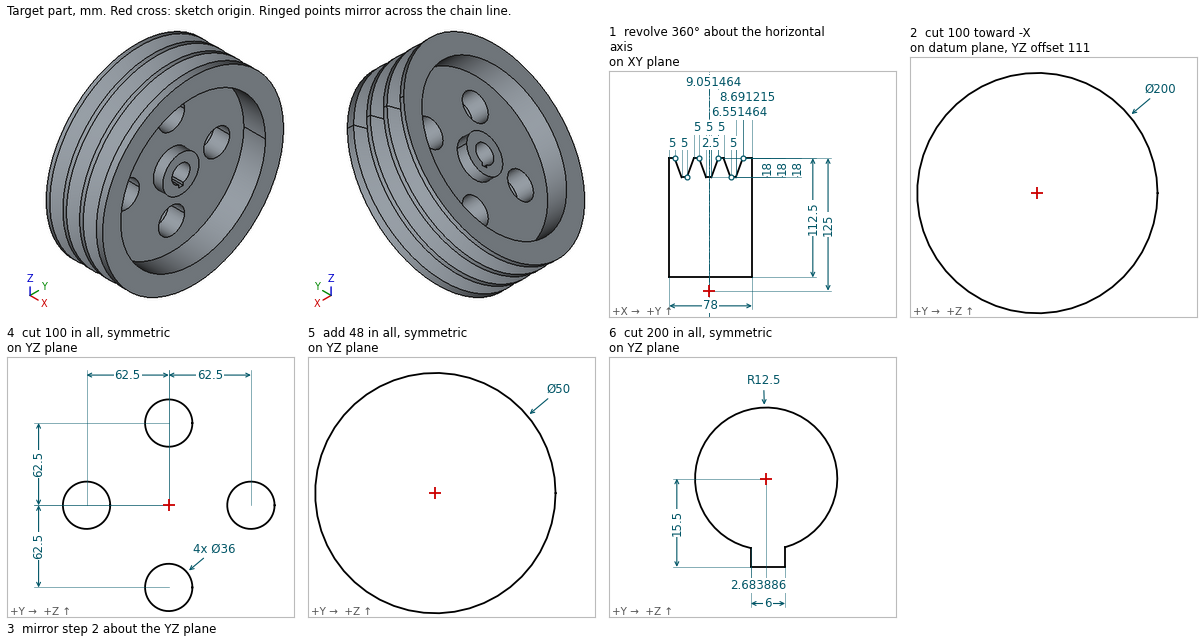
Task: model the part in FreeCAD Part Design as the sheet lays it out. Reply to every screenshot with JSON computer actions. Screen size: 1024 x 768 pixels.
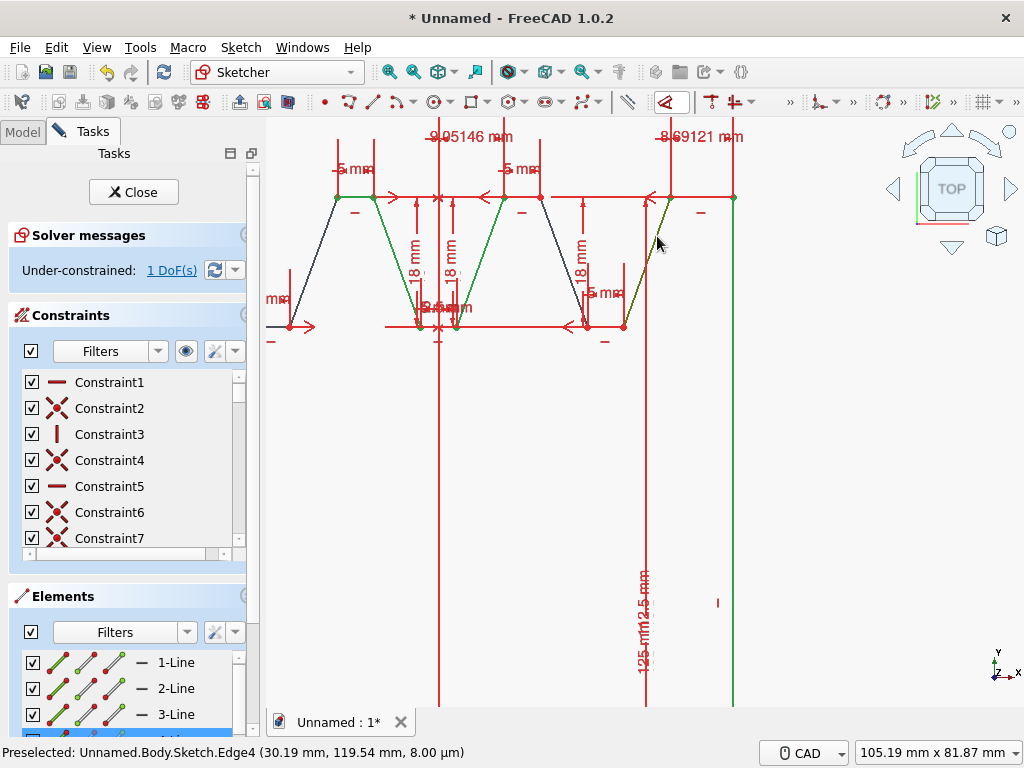
{"action": "left_click", "coordinate": [684, 102]}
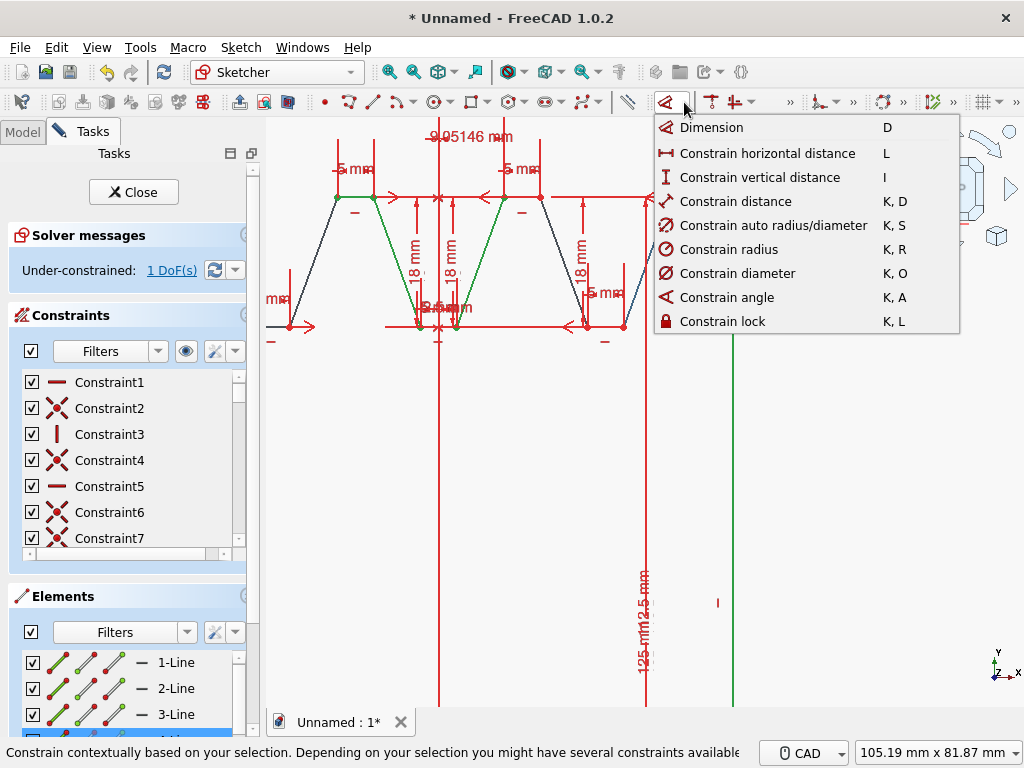
{"action": "left_click", "coordinate": [807, 153]}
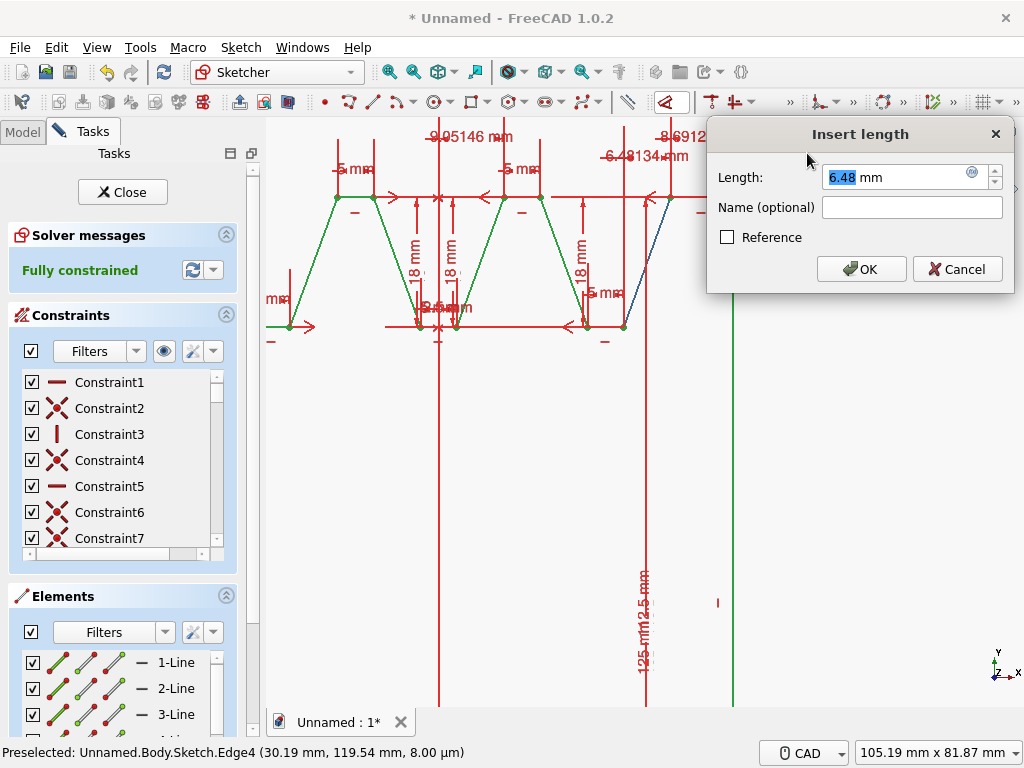
{"action": "type", "text": "6.551464"}
{"action": "key", "text": "Return"}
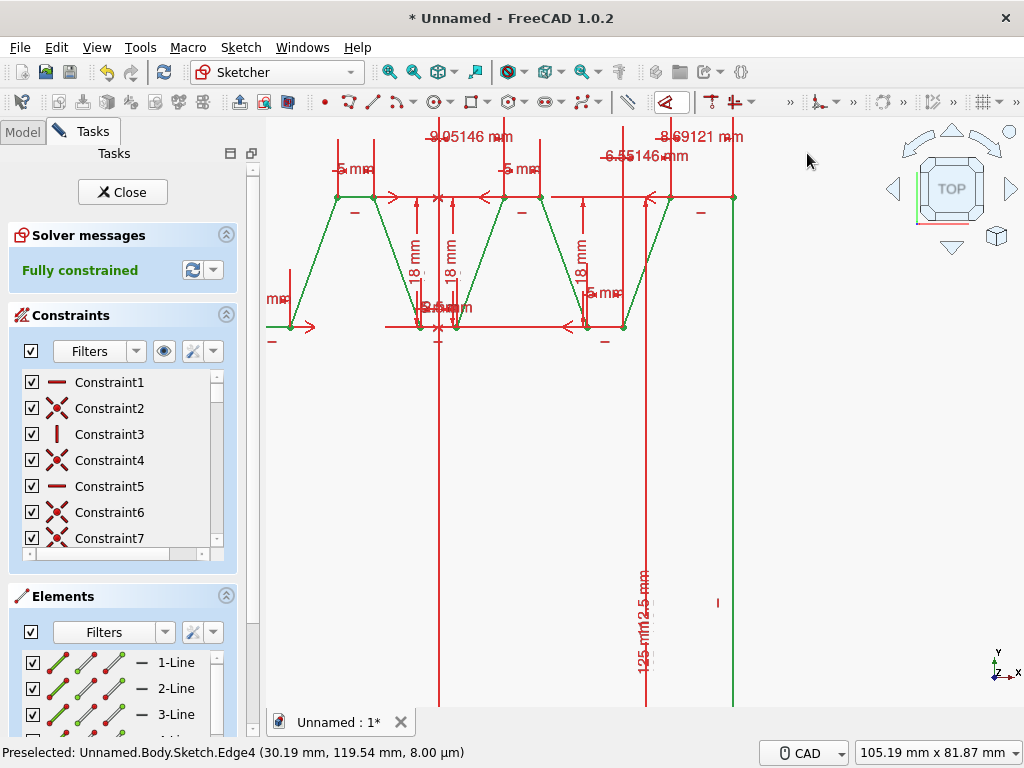
{"action": "left_click", "coordinate": [123, 192]}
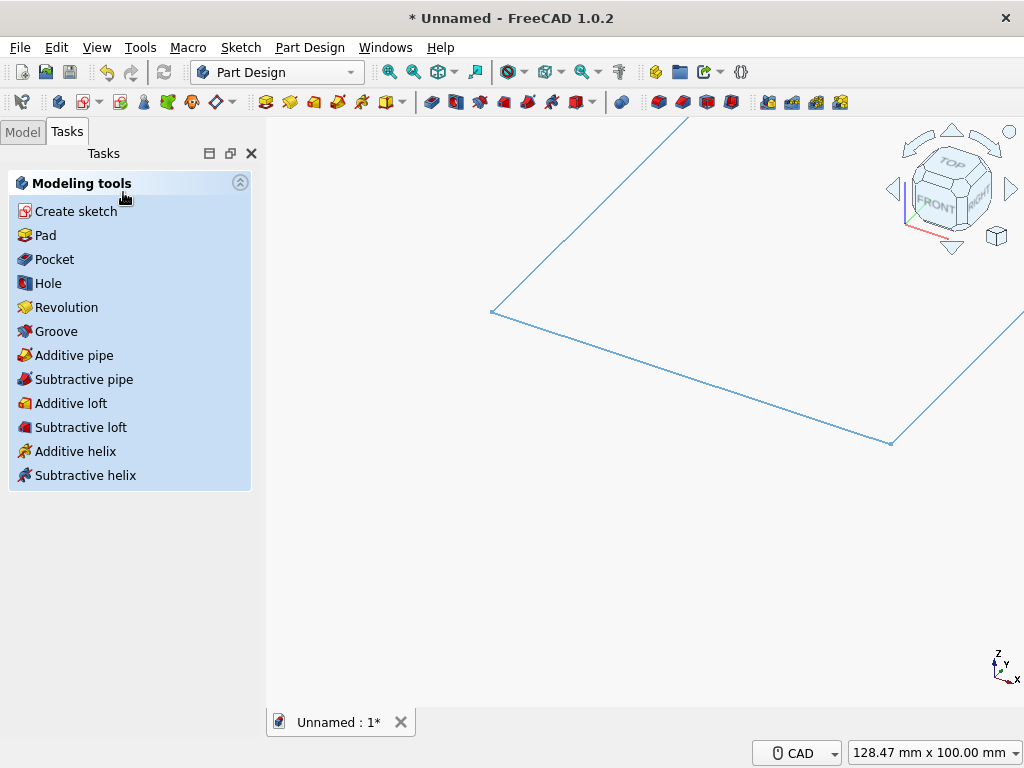
{"action": "left_click", "coordinate": [290, 102]}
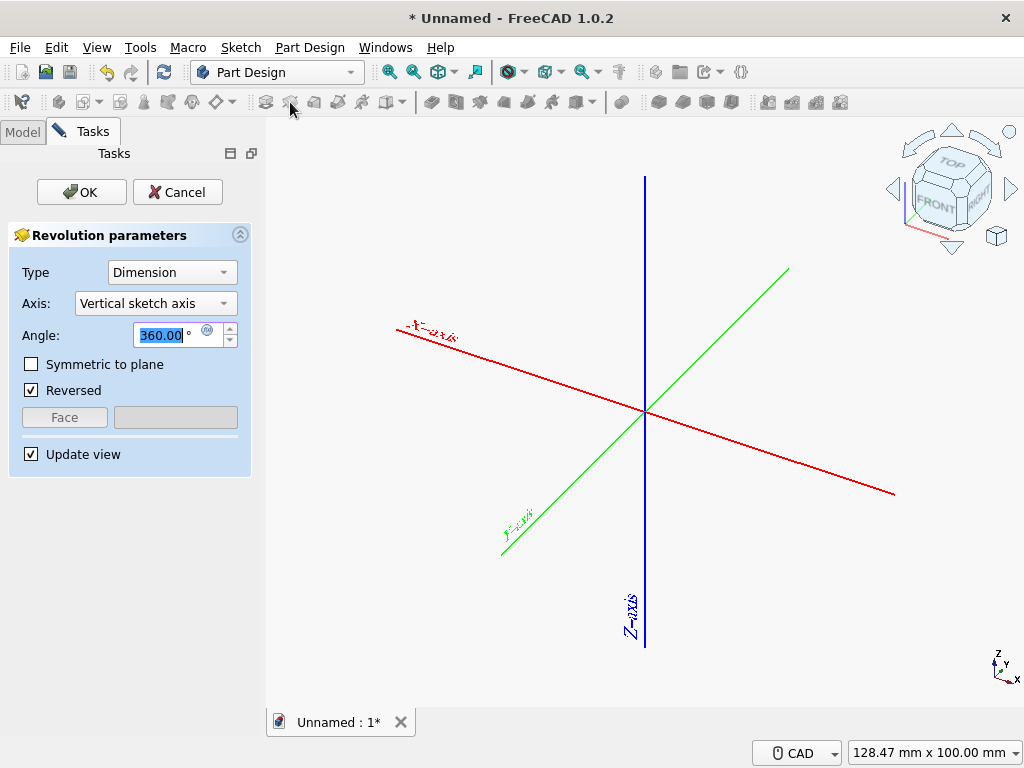
{"action": "left_click", "coordinate": [156, 304]}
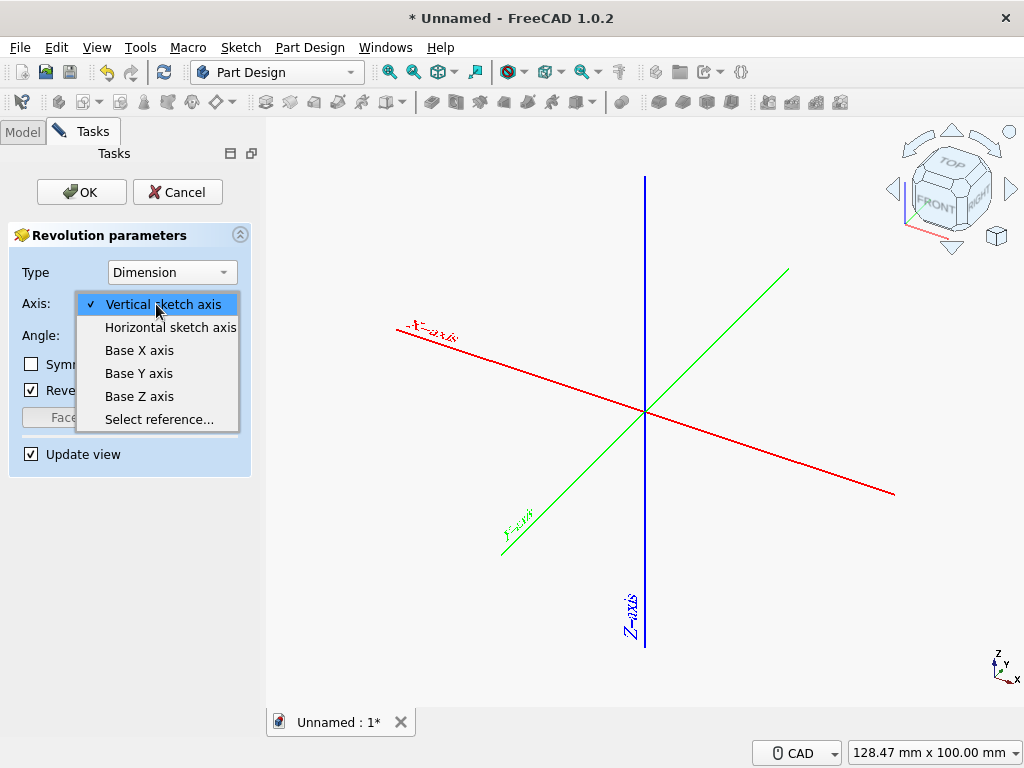
{"action": "left_click", "coordinate": [156, 328]}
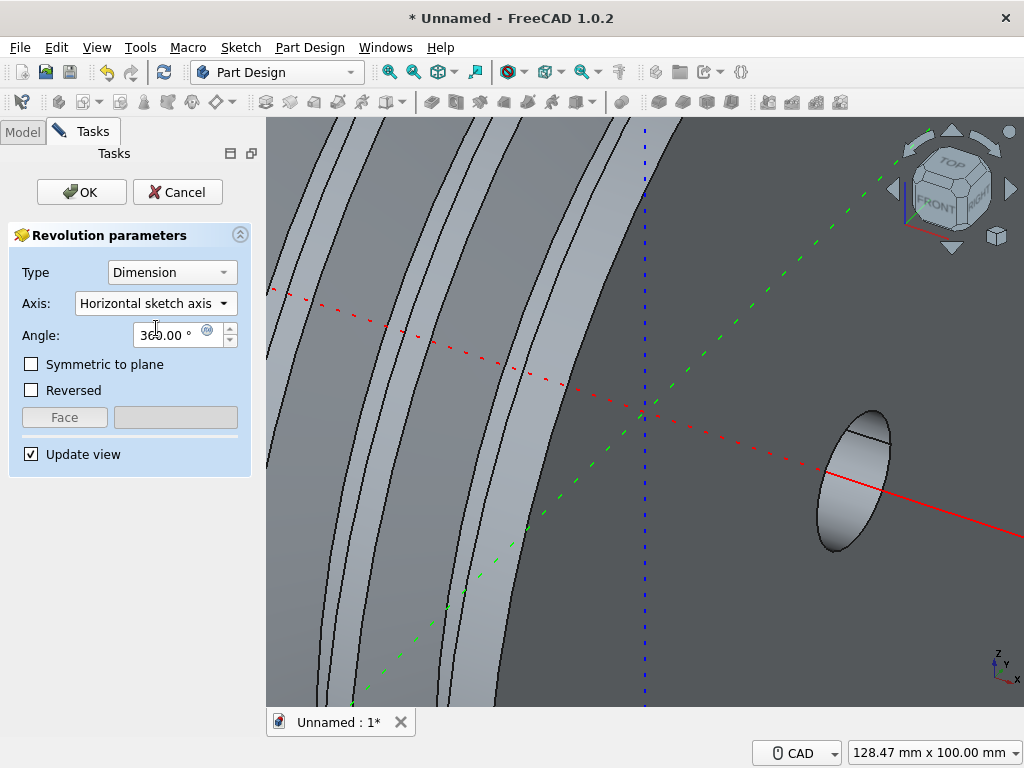
{"action": "left_click", "coordinate": [82, 192]}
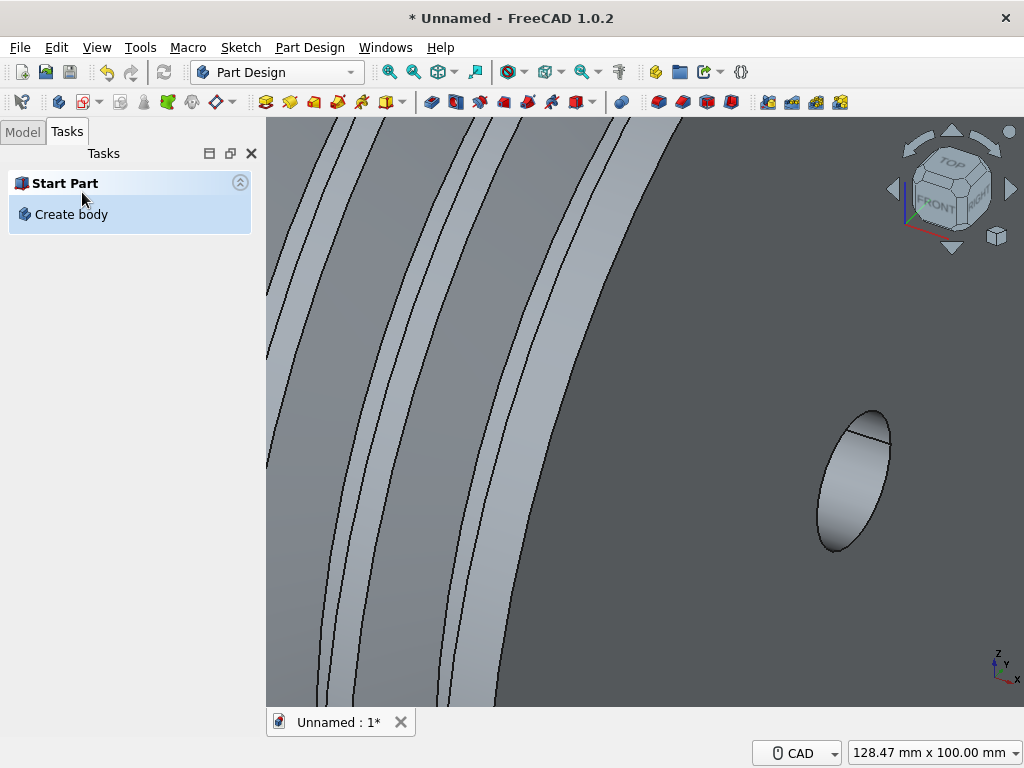
{"action": "left_click", "coordinate": [390, 72]}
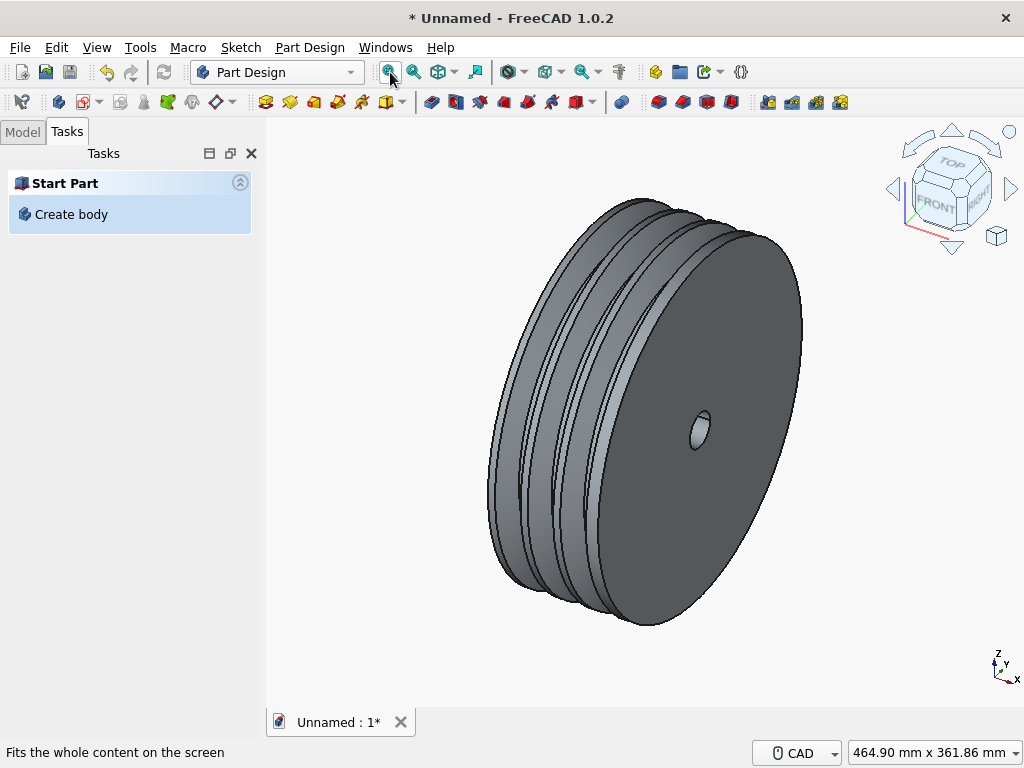
{"action": "left_click", "coordinate": [23, 131]}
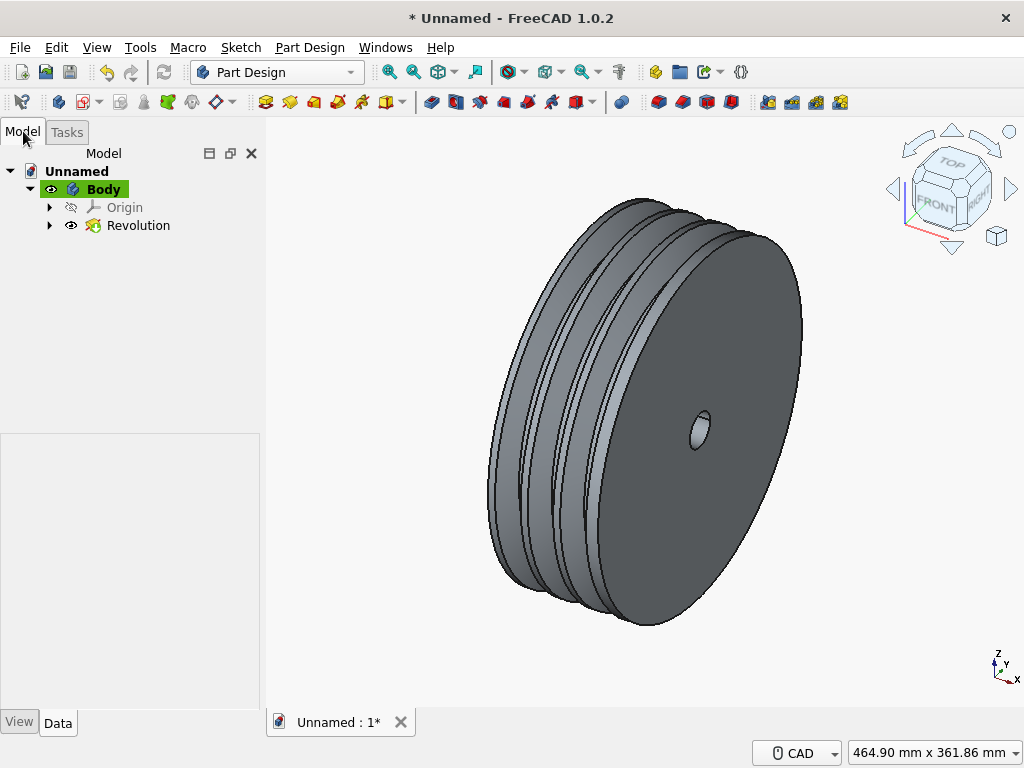
{"action": "left_click", "coordinate": [50, 207]}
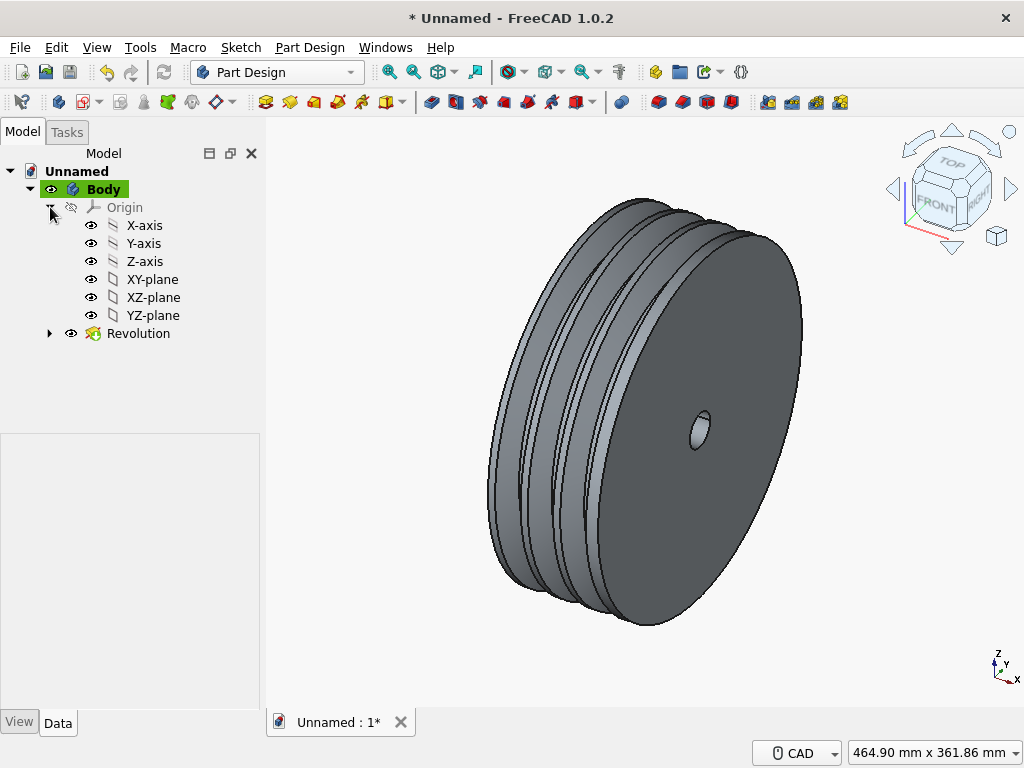
{"action": "left_click", "coordinate": [136, 315]}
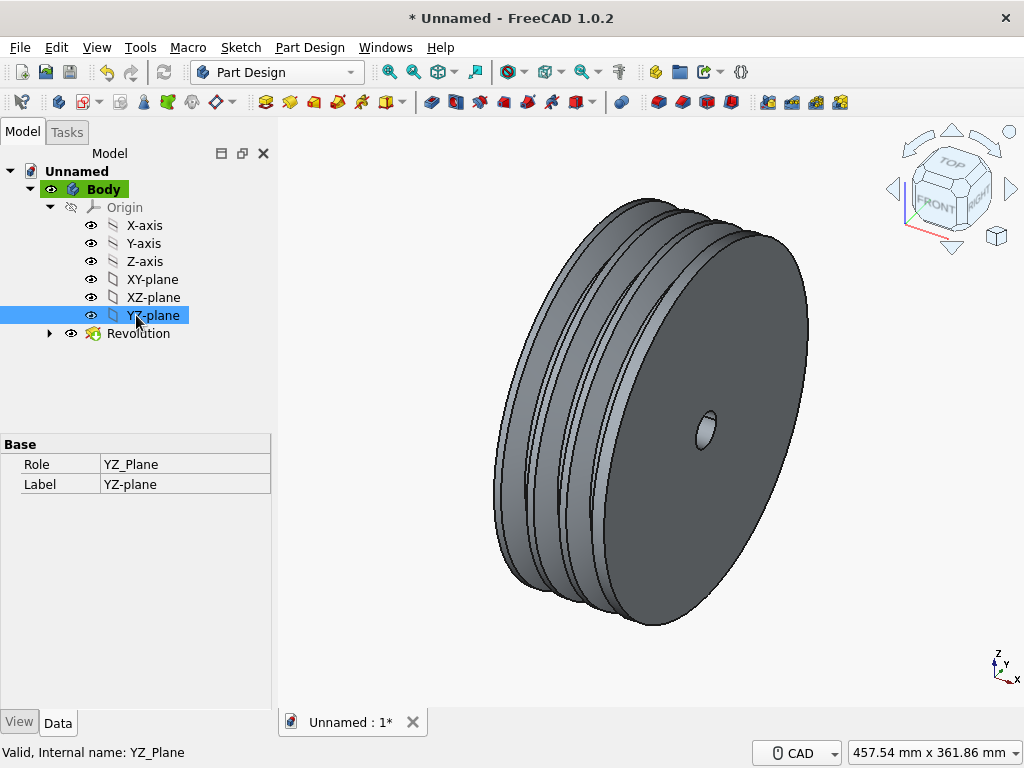
{"action": "left_click", "coordinate": [216, 102]}